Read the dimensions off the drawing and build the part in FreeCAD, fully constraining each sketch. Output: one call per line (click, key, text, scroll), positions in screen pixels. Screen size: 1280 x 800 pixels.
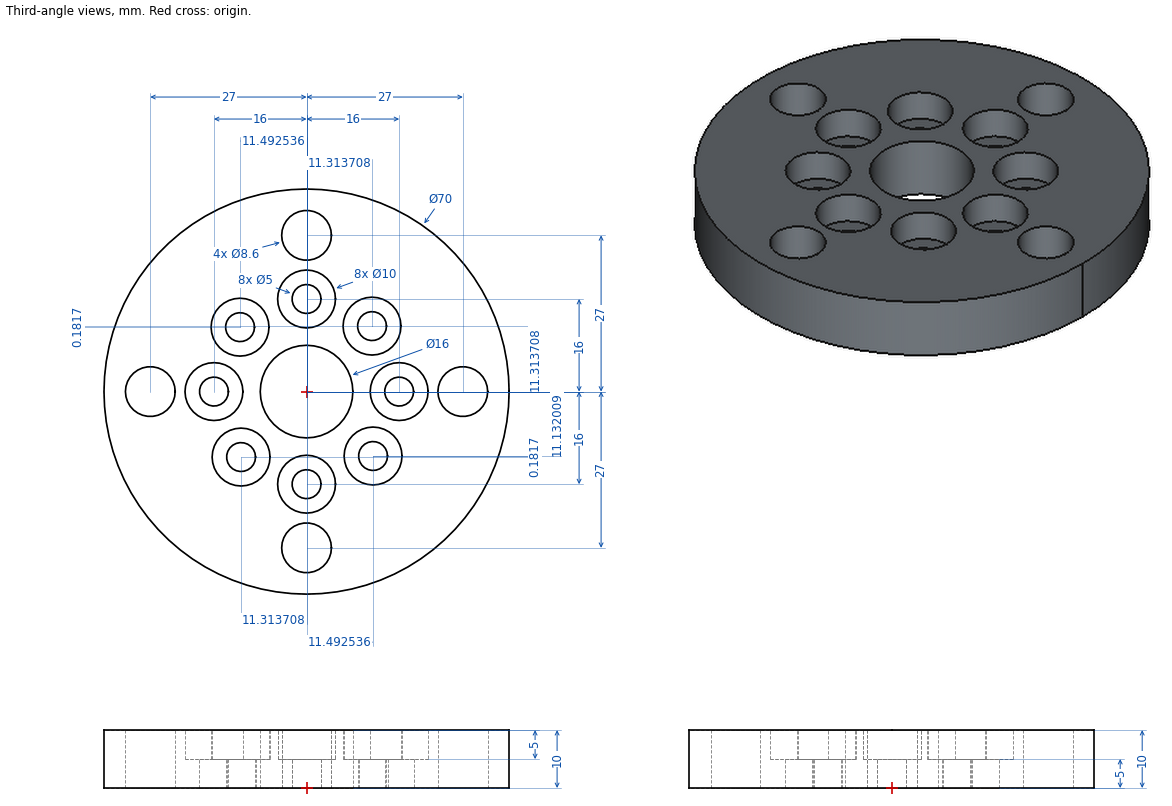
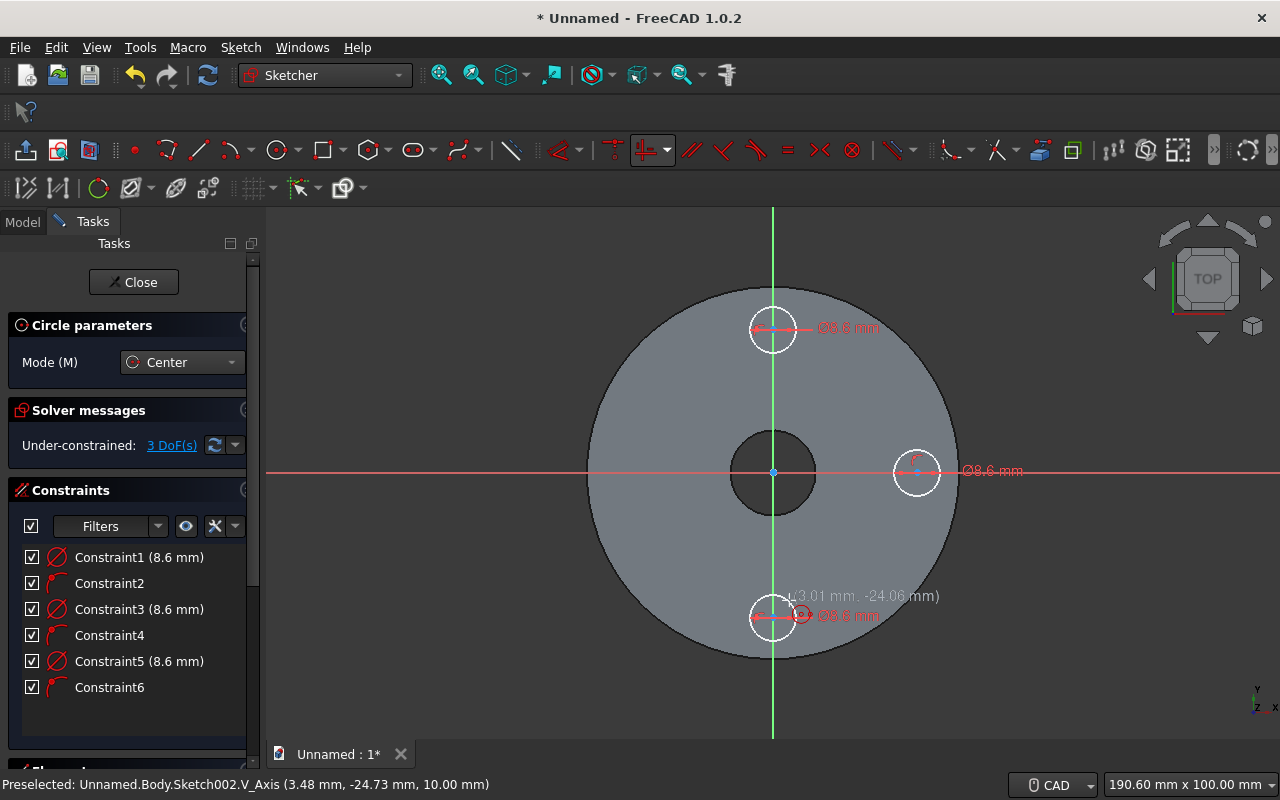
click(629, 473)
move(646, 457)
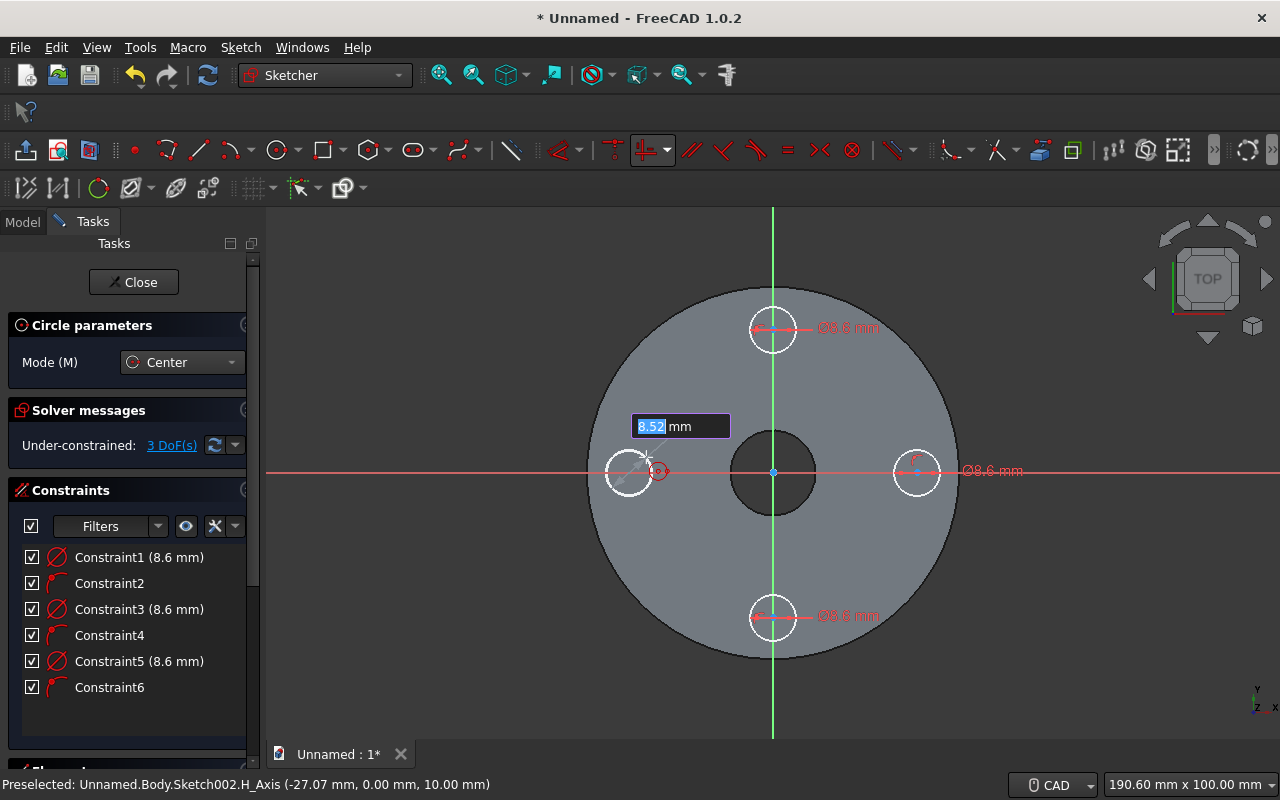
text(8.6)
key(Return)
key(Escape)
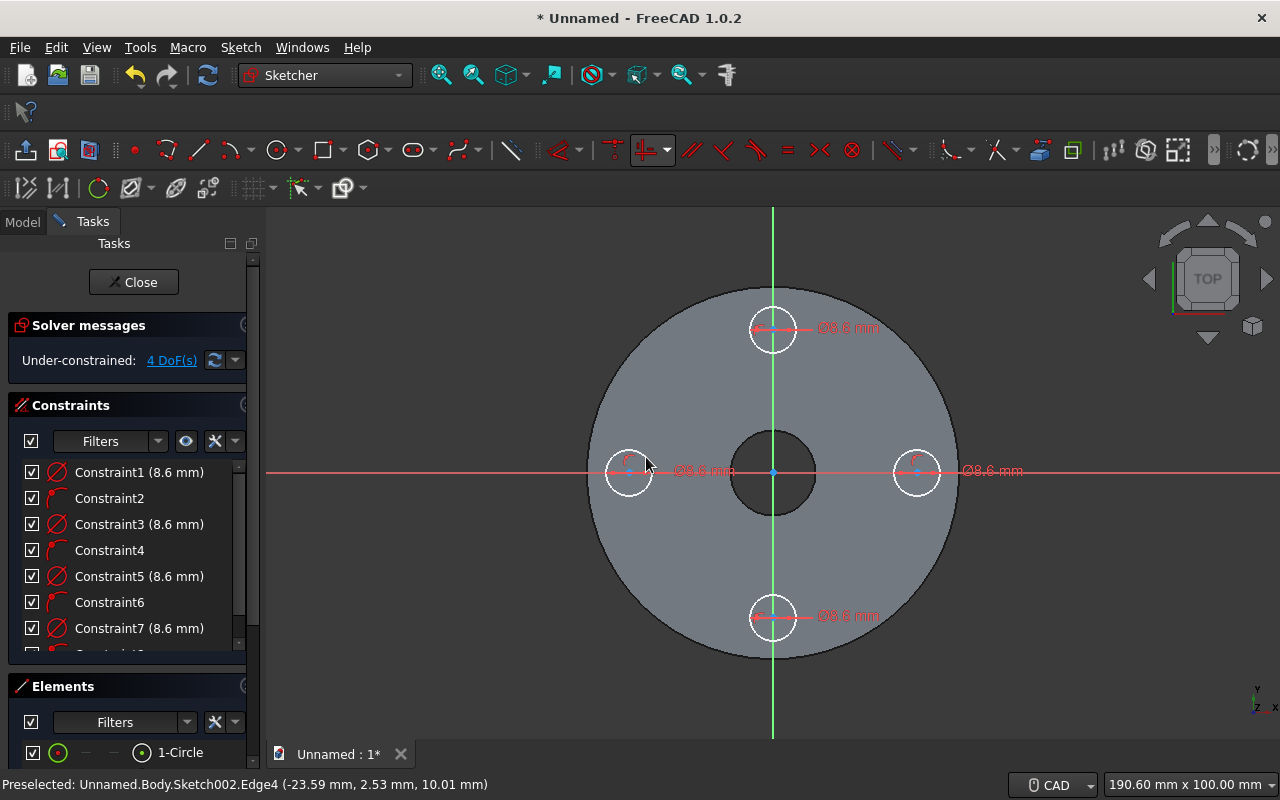
click(558, 150)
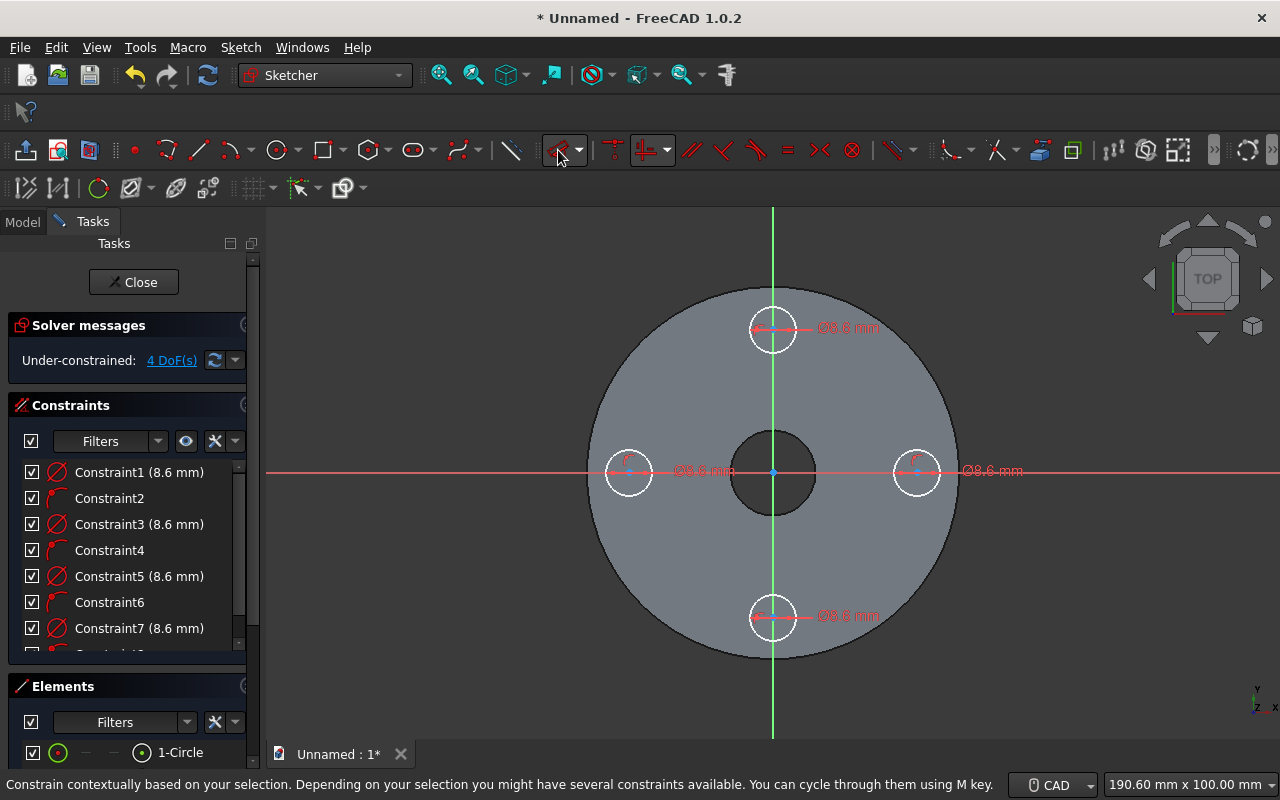
click(773, 330)
click(807, 402)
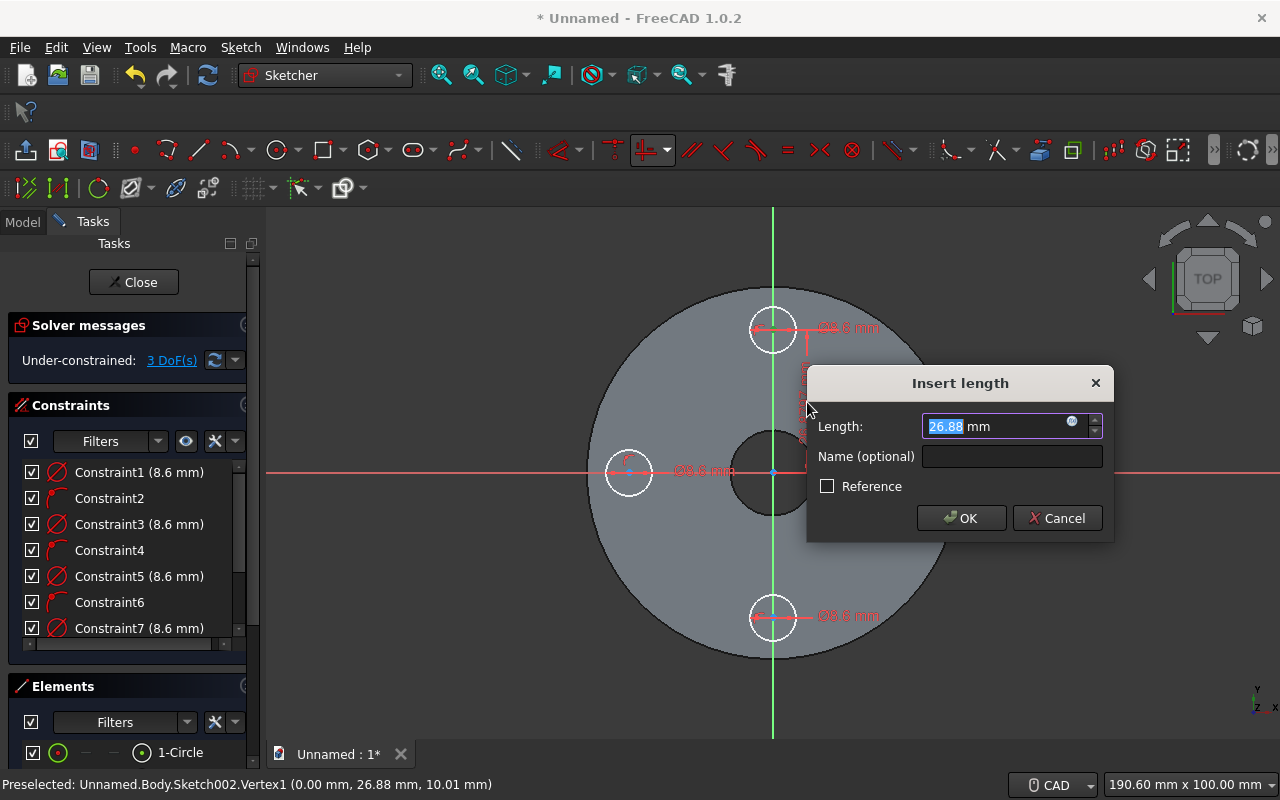
text(27)
key(Return)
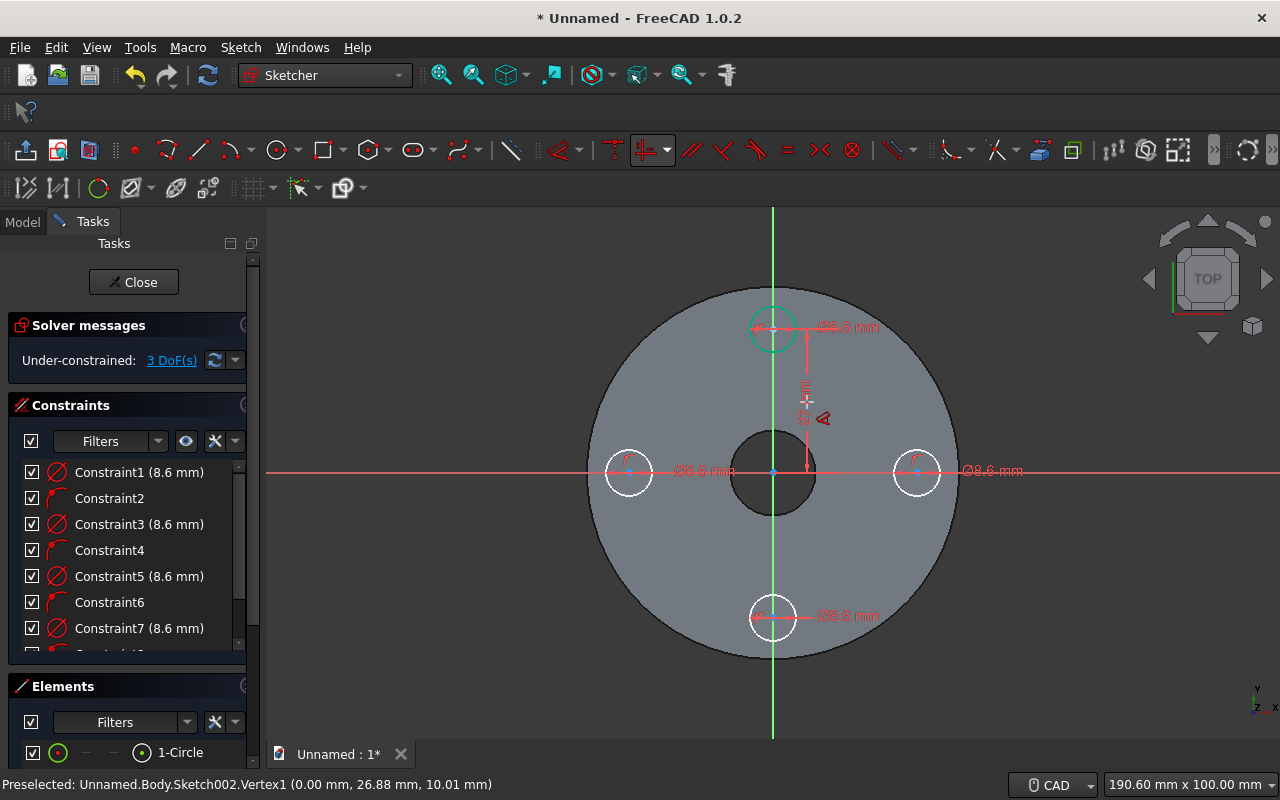
click(917, 473)
click(845, 507)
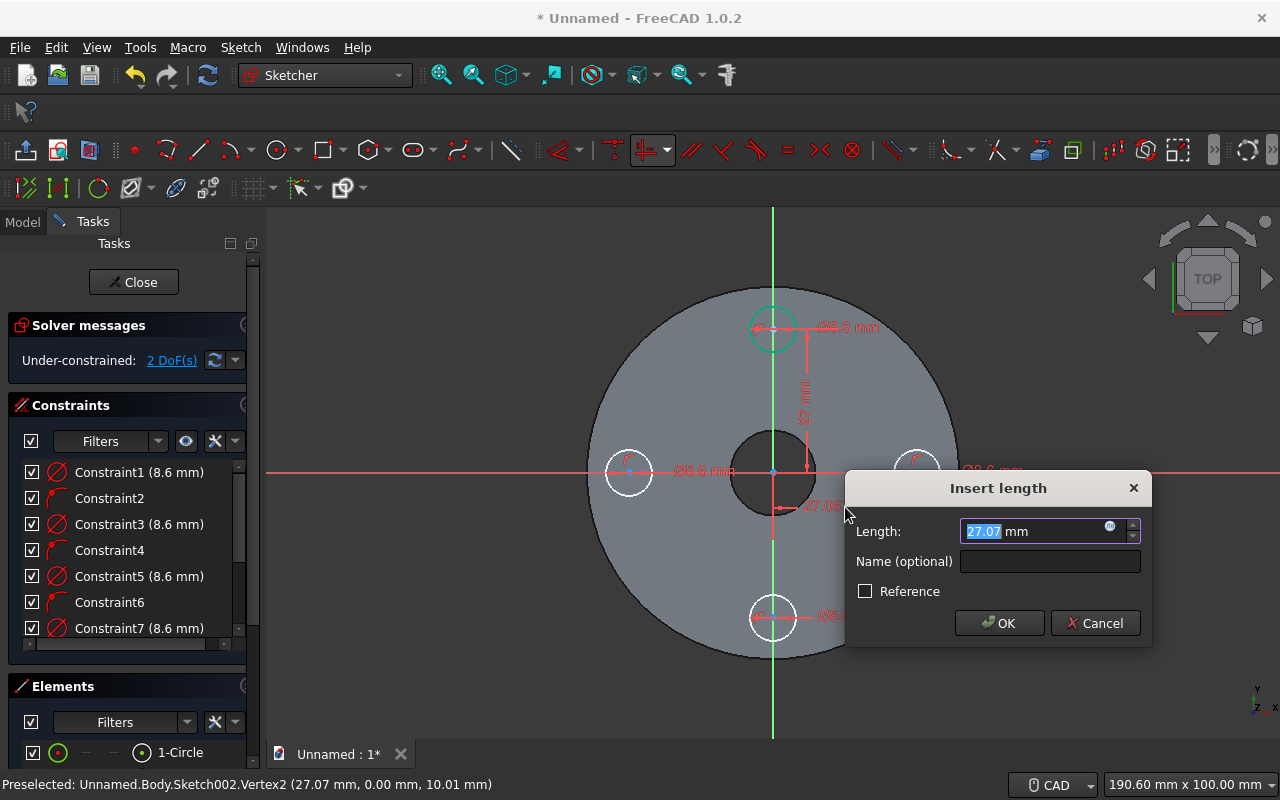
text(27)
key(Return)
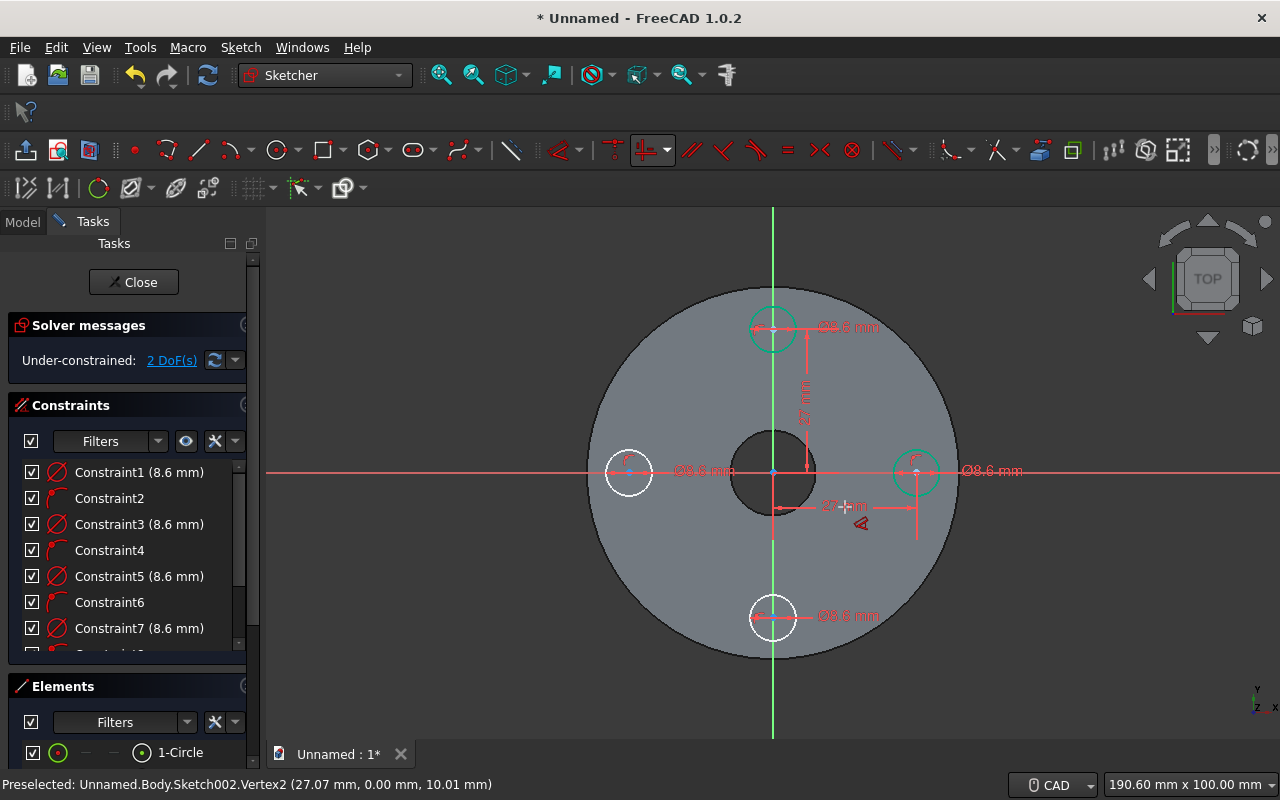
click(773, 618)
click(807, 546)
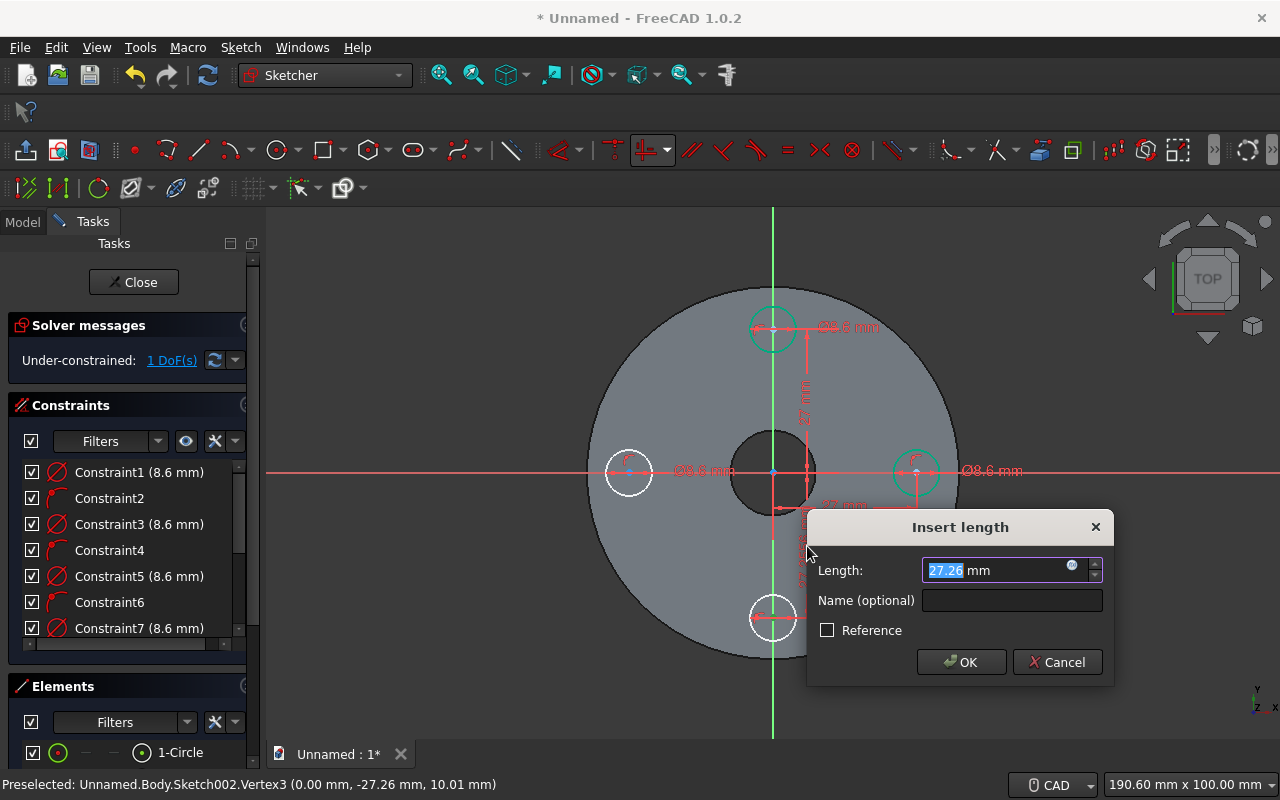
text(27)
key(Return)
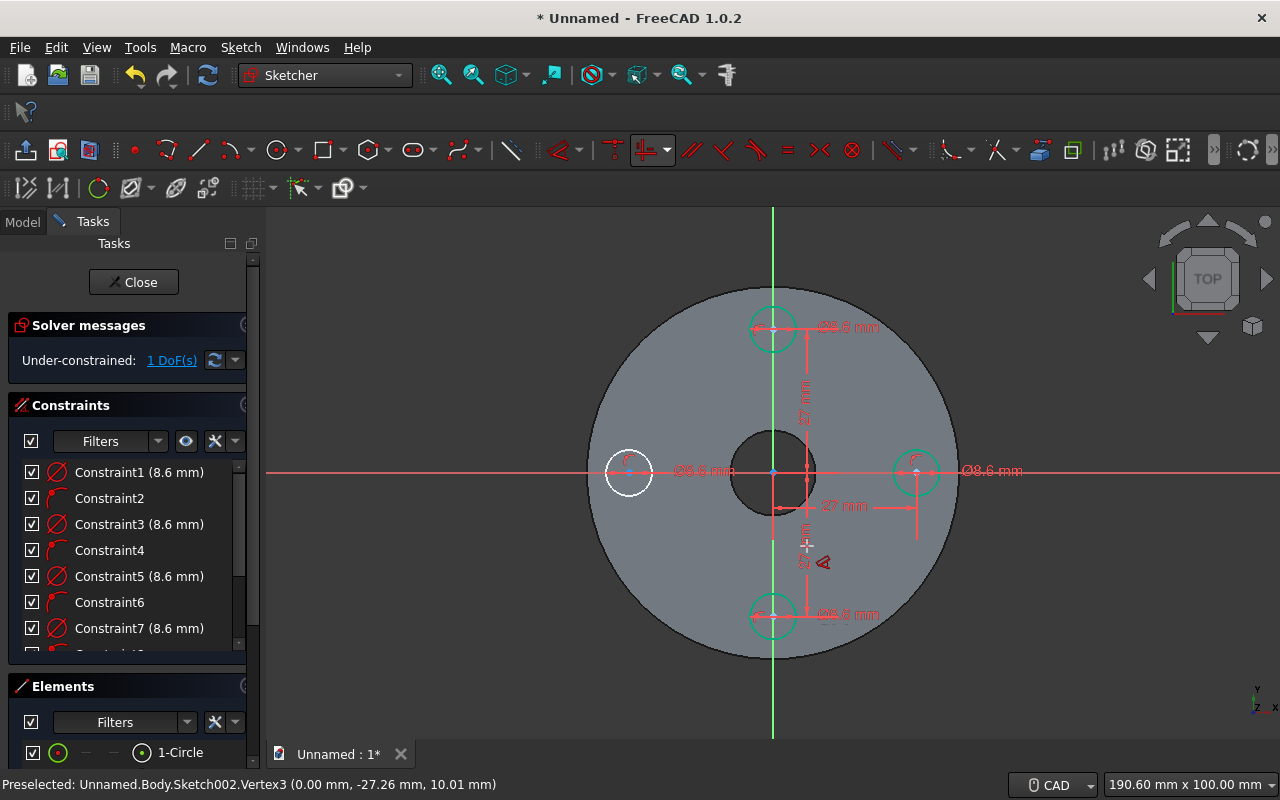
click(629, 473)
click(701, 507)